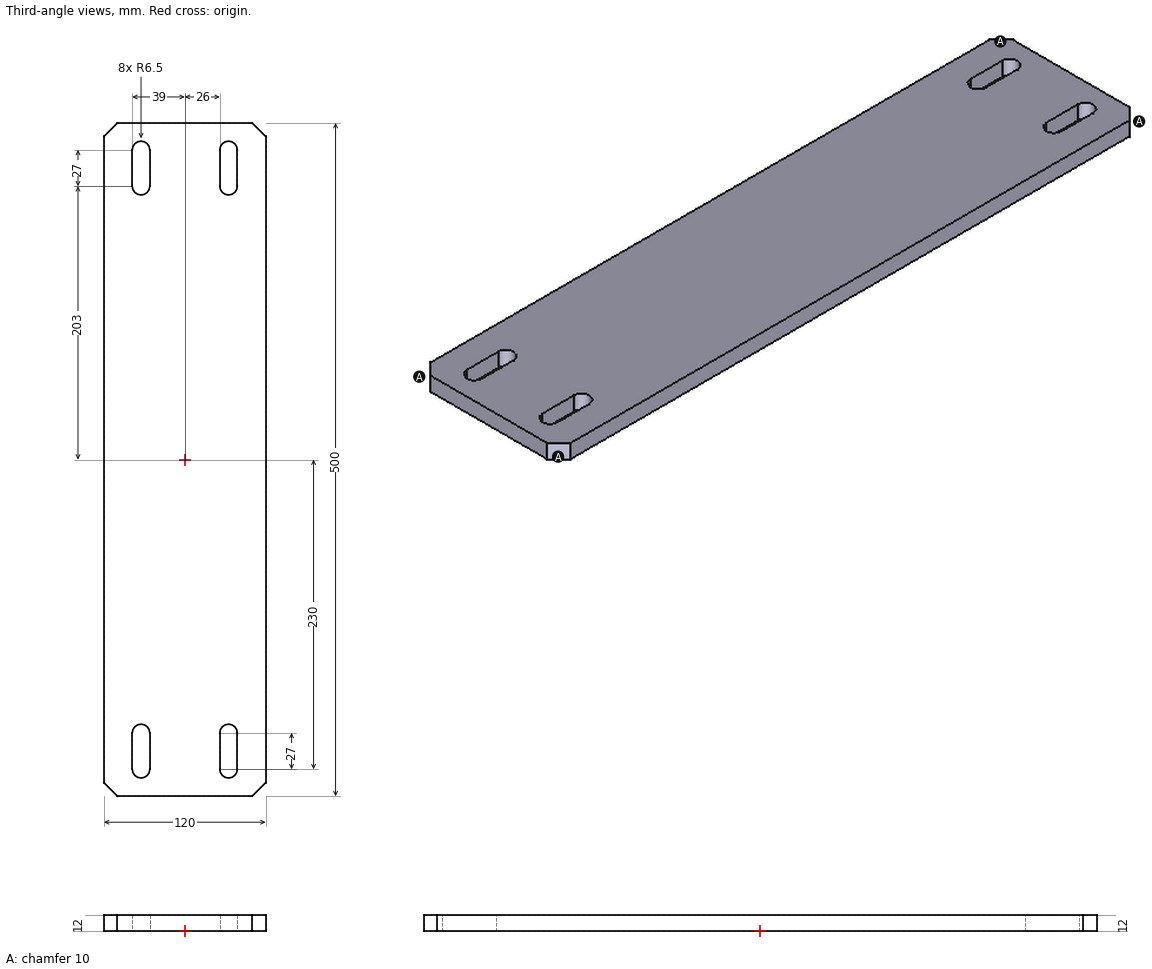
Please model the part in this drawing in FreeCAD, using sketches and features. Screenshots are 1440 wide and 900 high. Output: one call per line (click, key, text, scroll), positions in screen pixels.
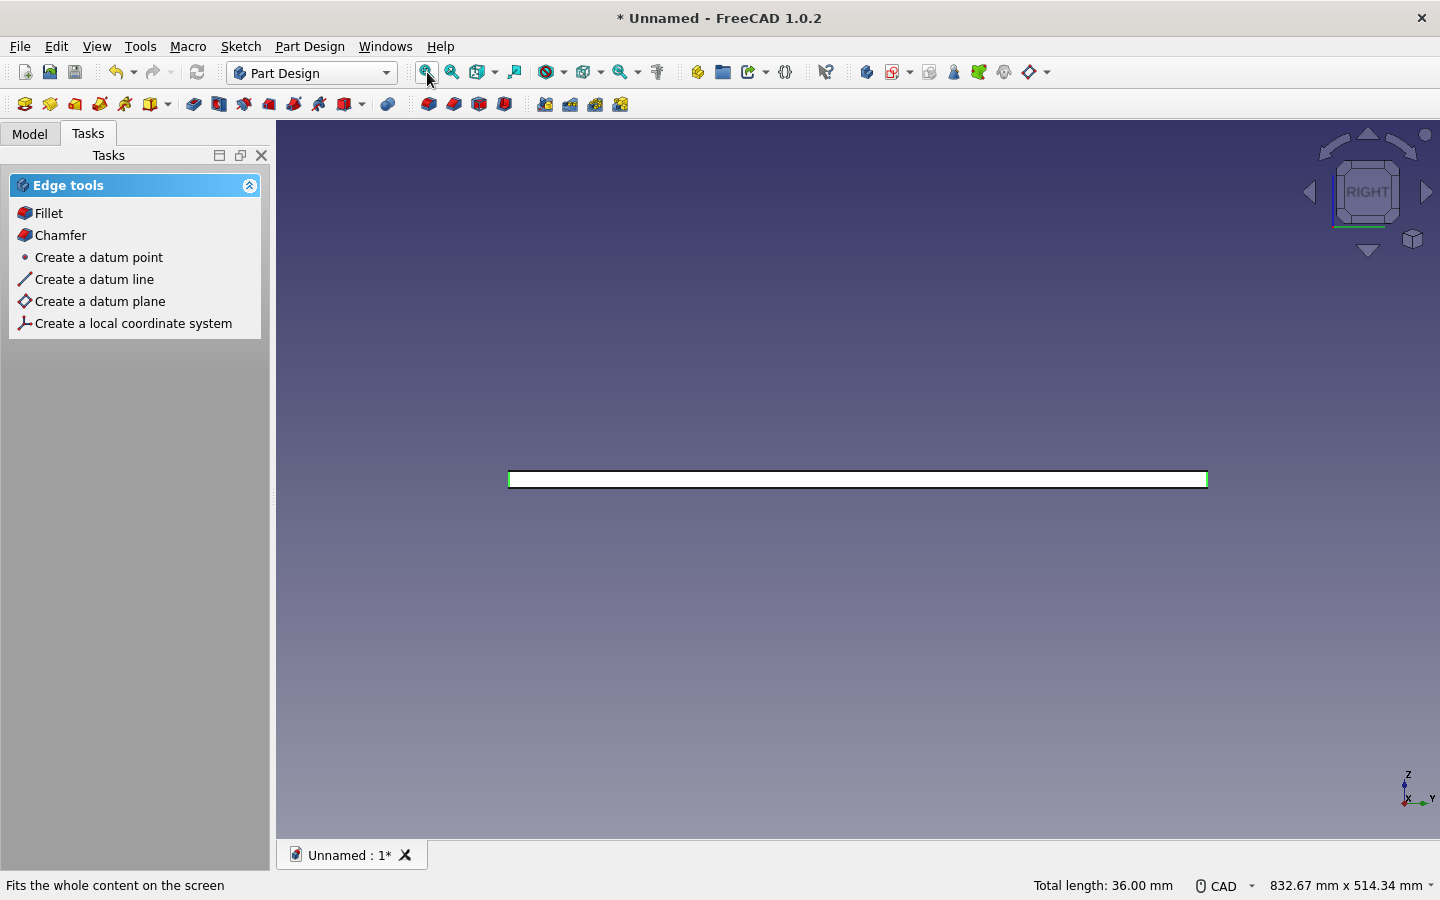
key(5)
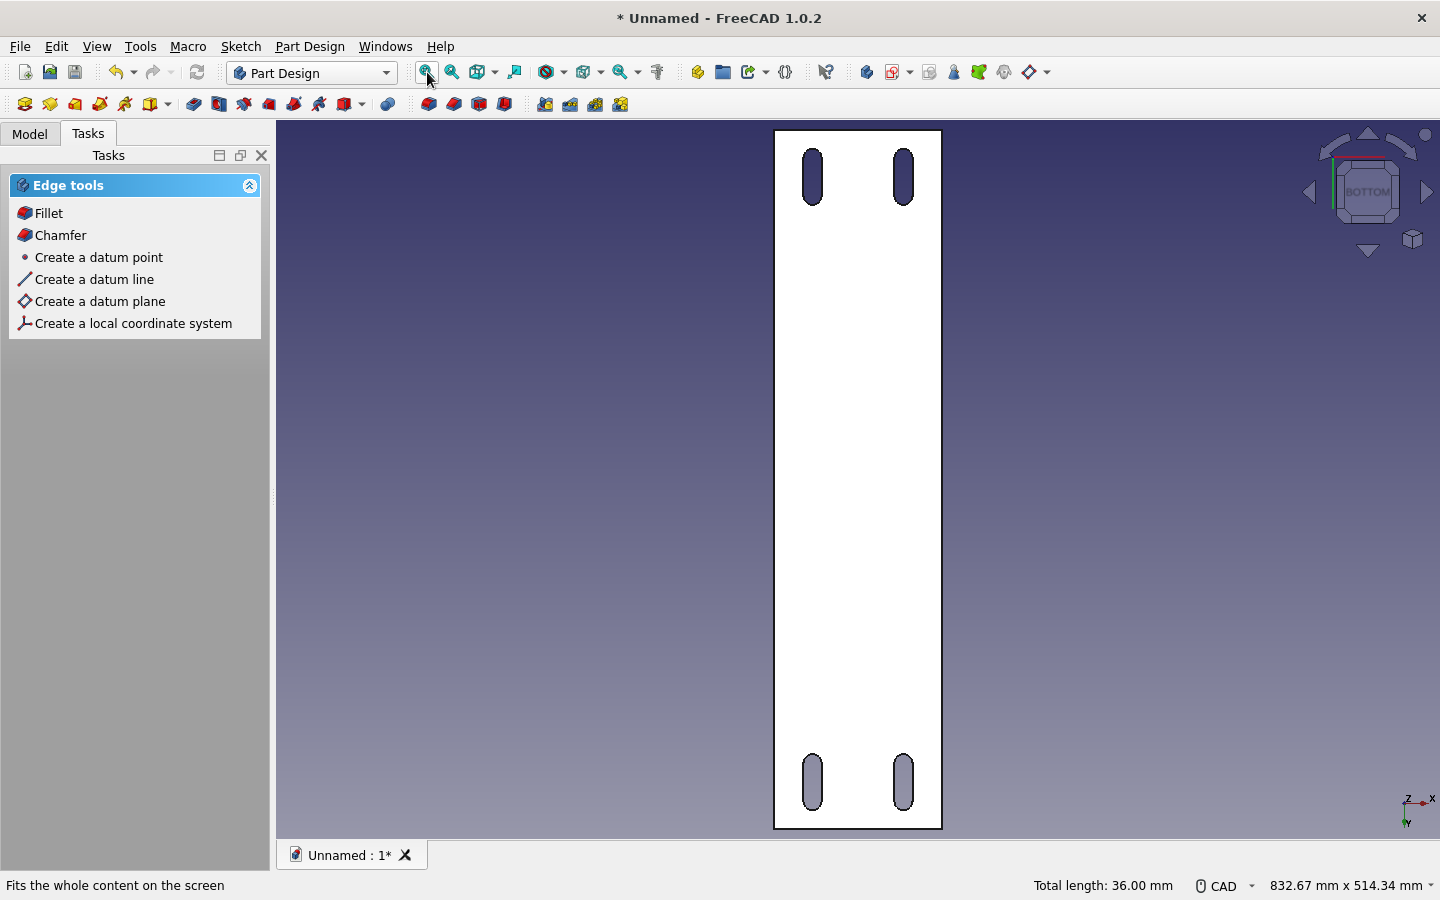
key(4)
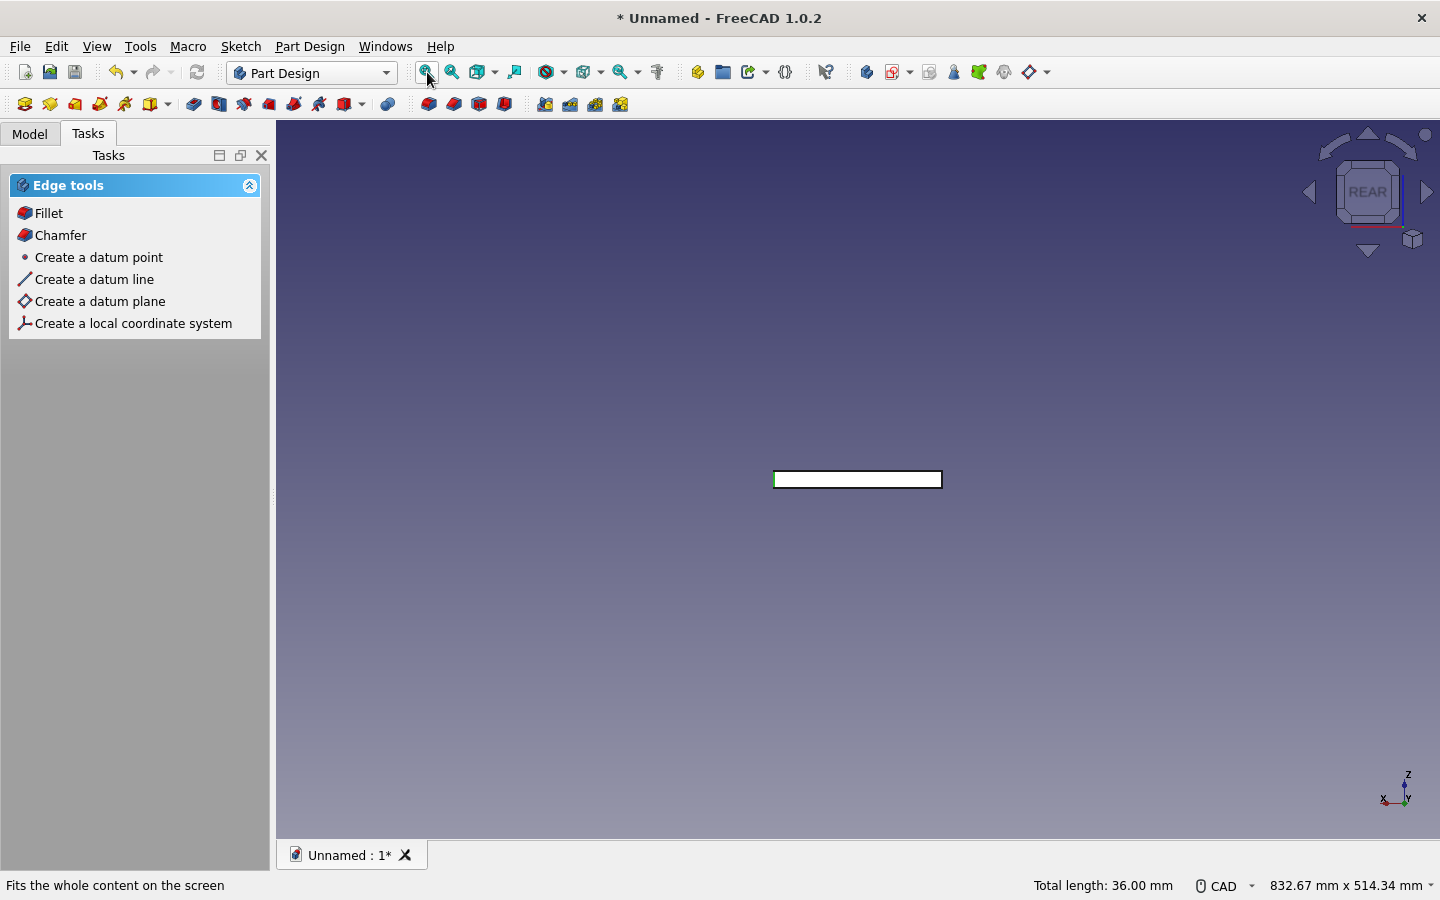
key(v)
key(f)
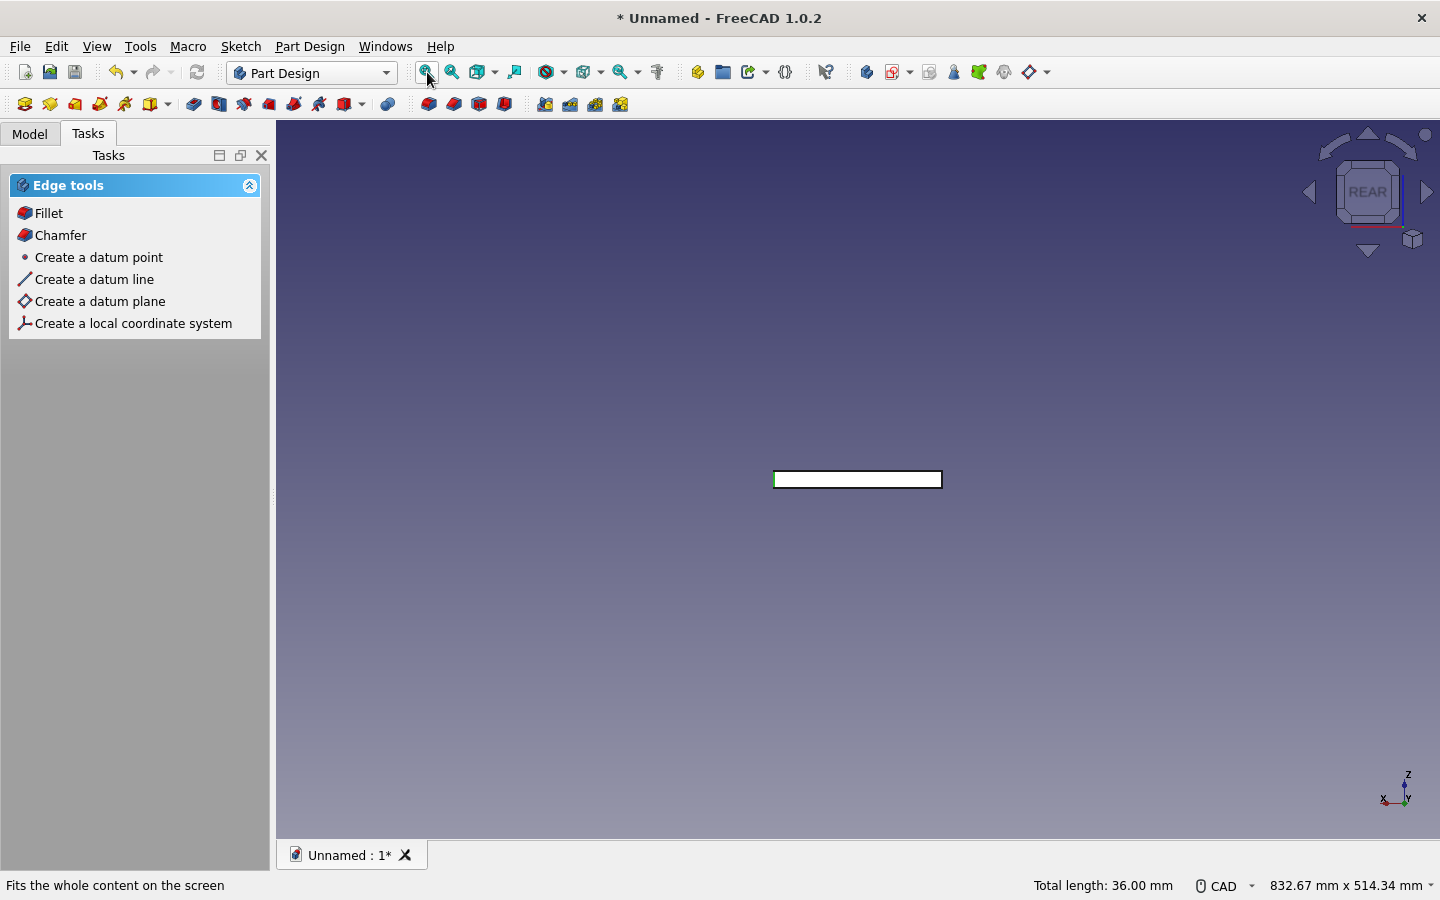
click(942, 479, ctrl)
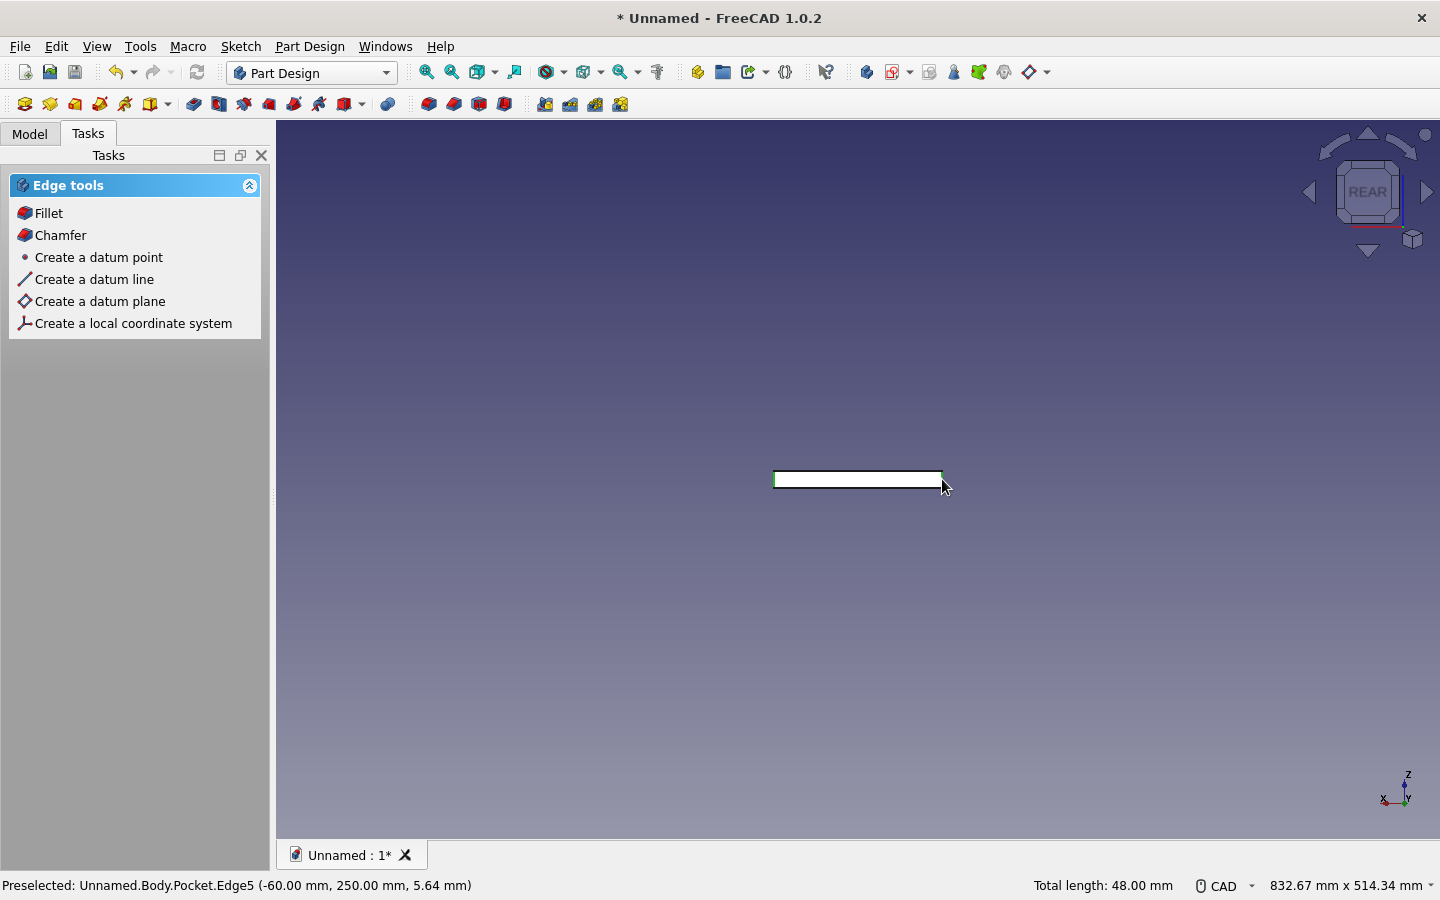
click(454, 104)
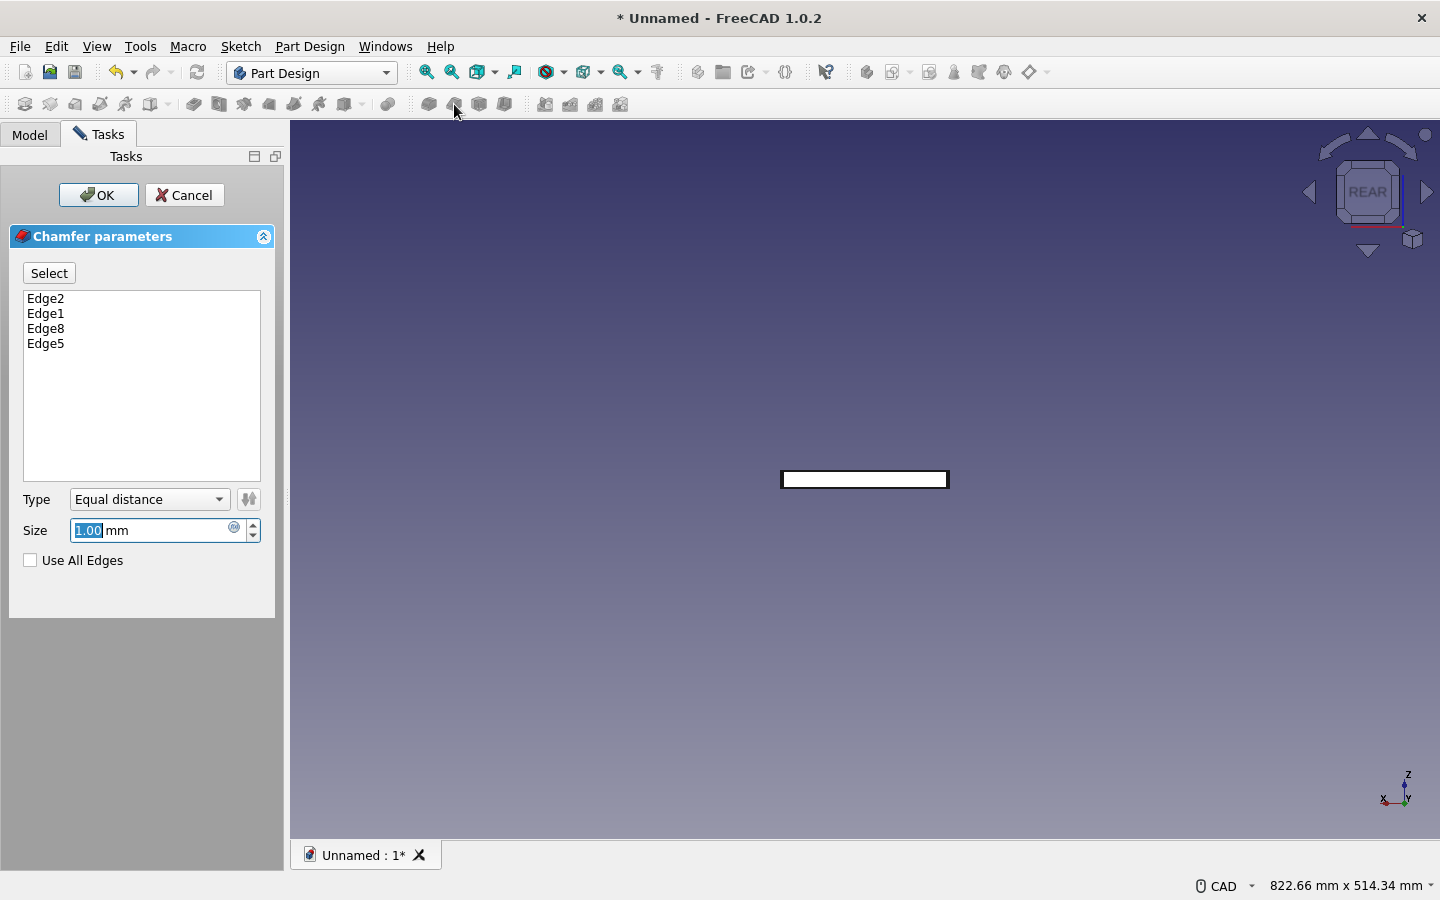
text(10)
key(Tab)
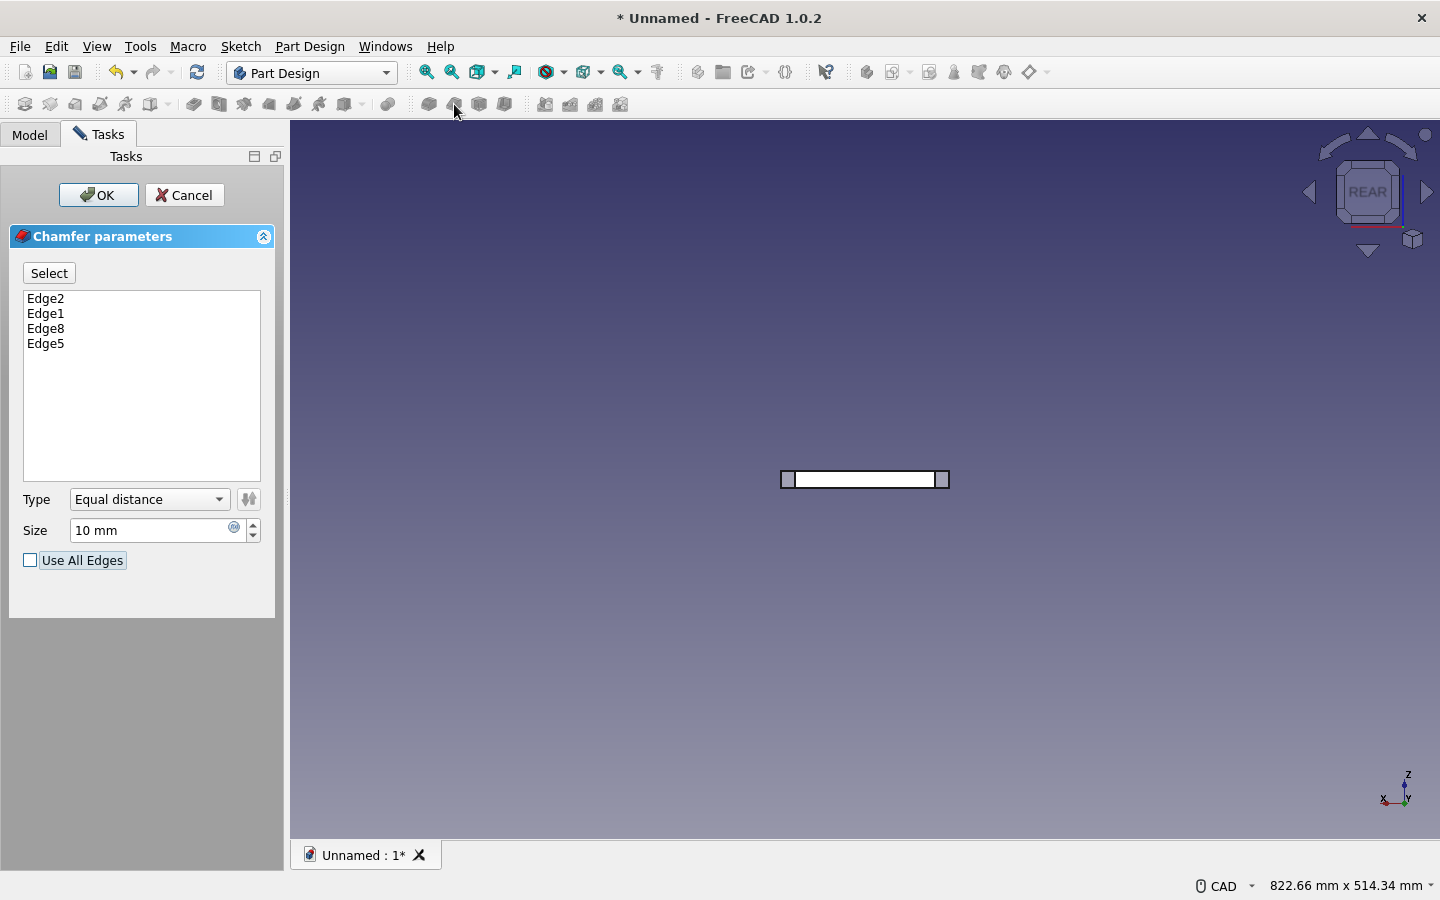
click(99, 195)